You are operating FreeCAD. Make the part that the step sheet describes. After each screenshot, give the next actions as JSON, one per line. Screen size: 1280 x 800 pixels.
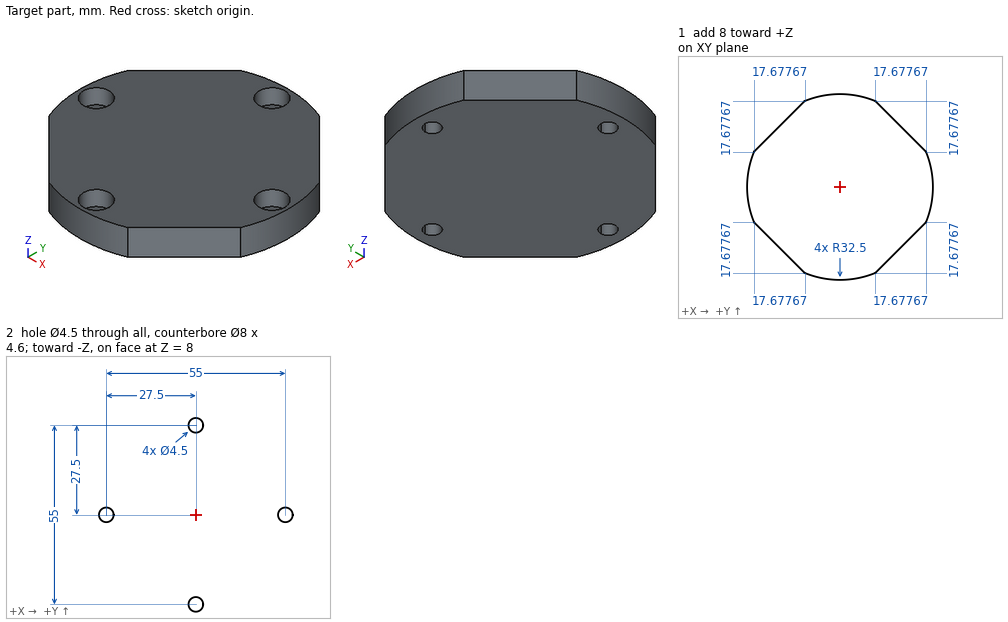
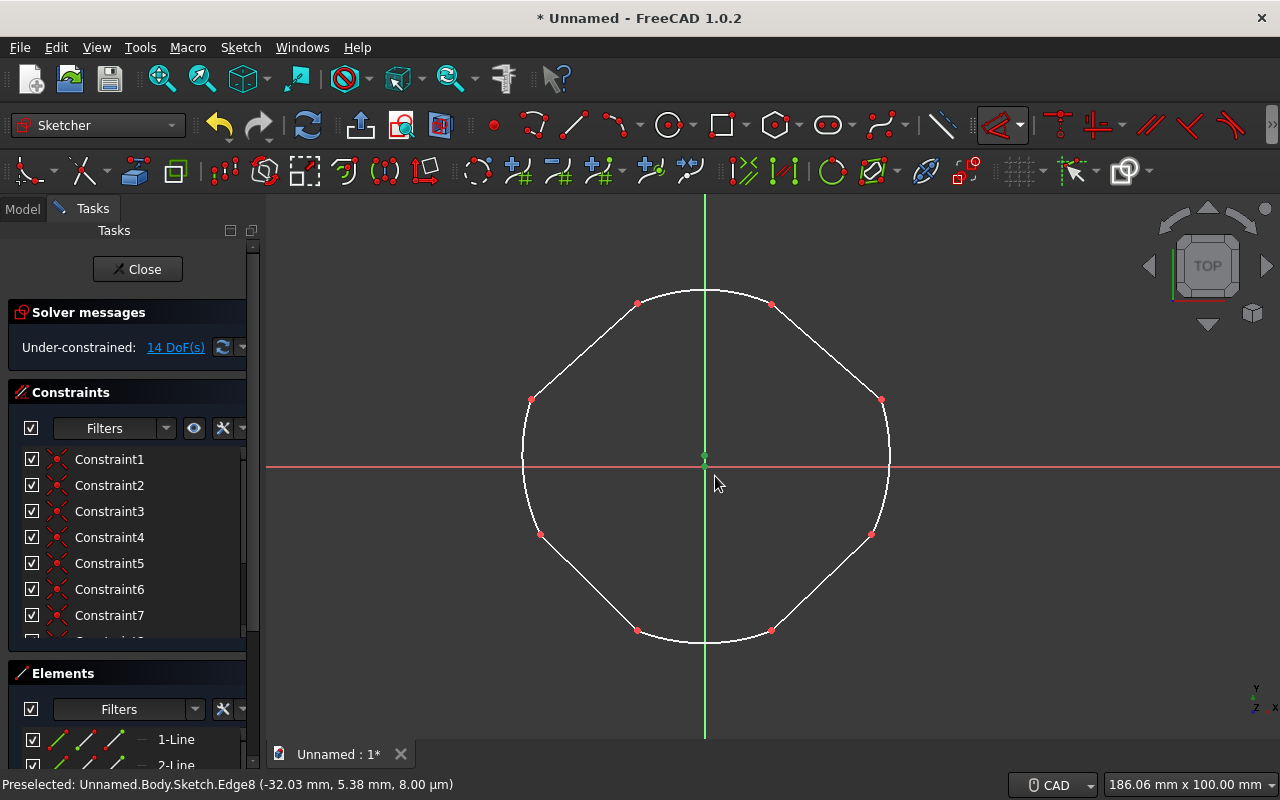
{"action": "left_click", "coordinate": [1058, 126]}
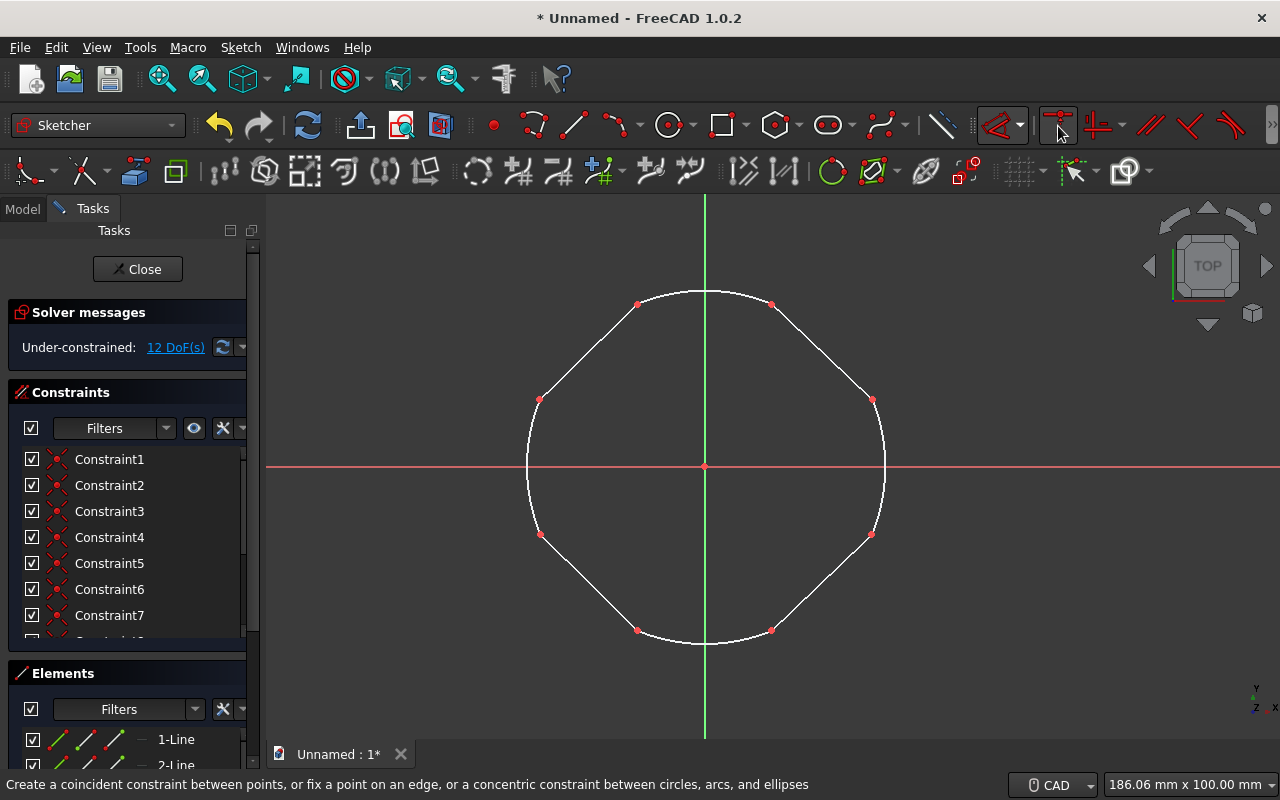
{"action": "left_click", "coordinate": [677, 642]}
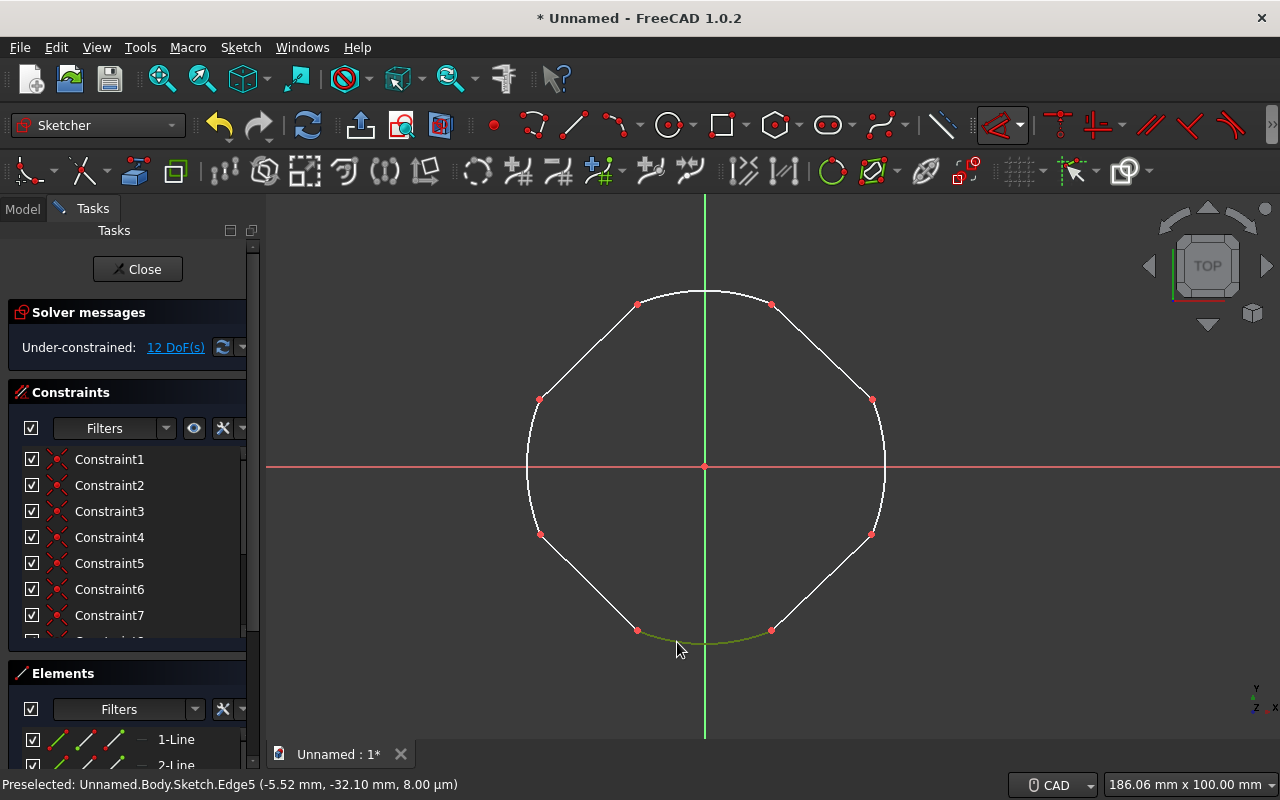
{"action": "left_click", "coordinate": [883, 495]}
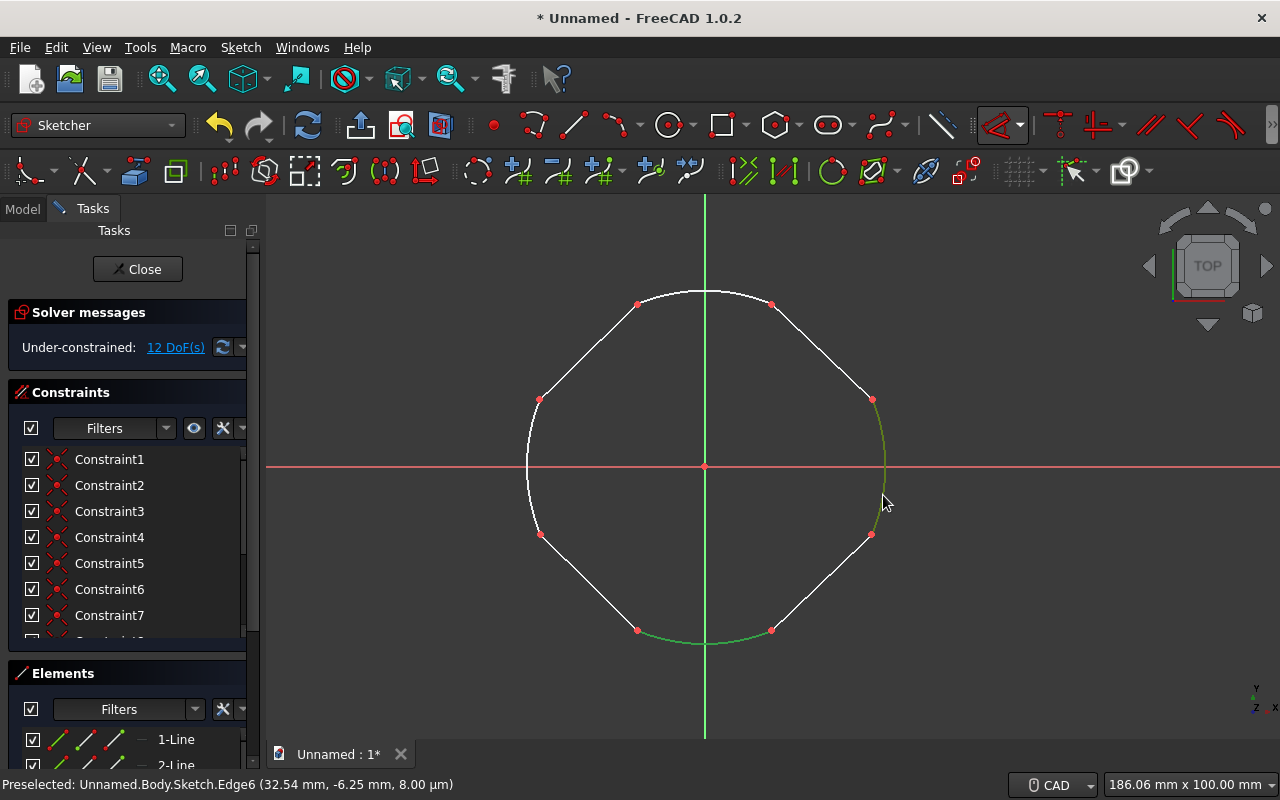
{"action": "left_click", "coordinate": [732, 293]}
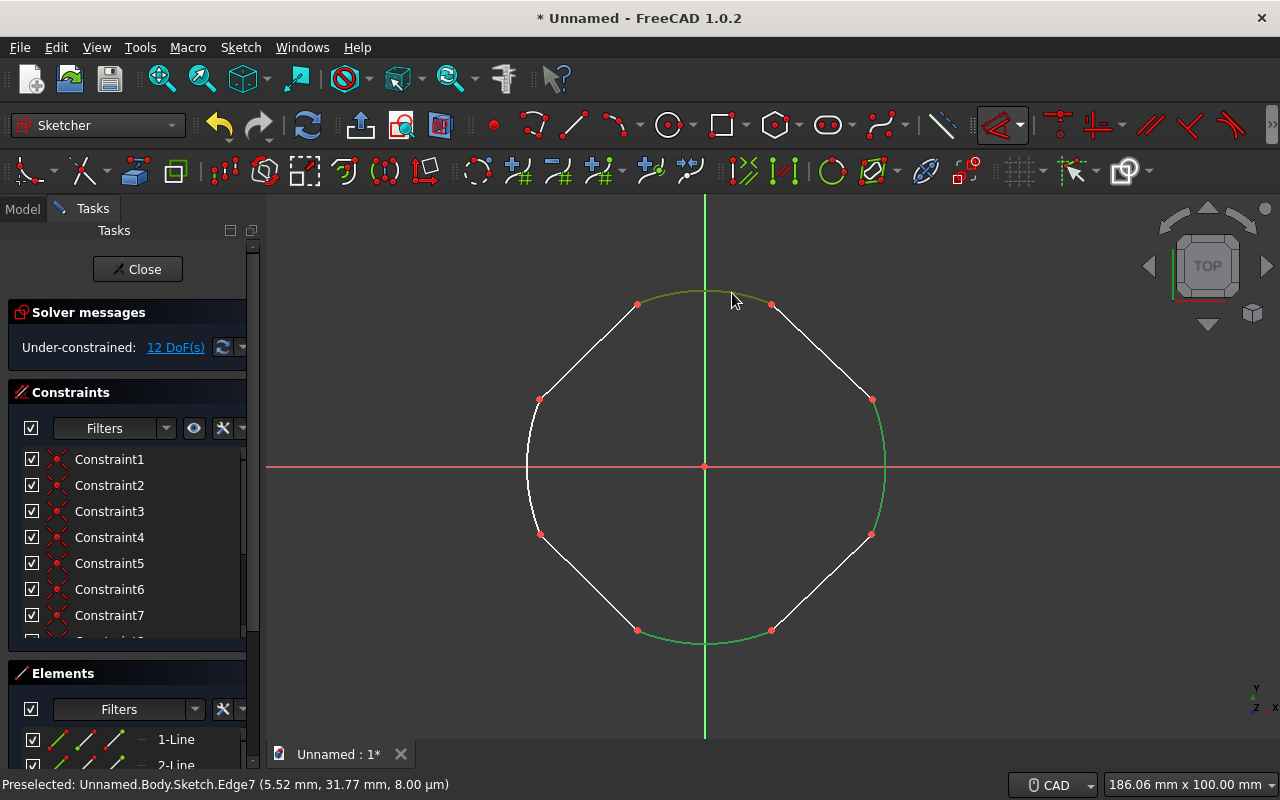
{"action": "left_click", "coordinate": [529, 440]}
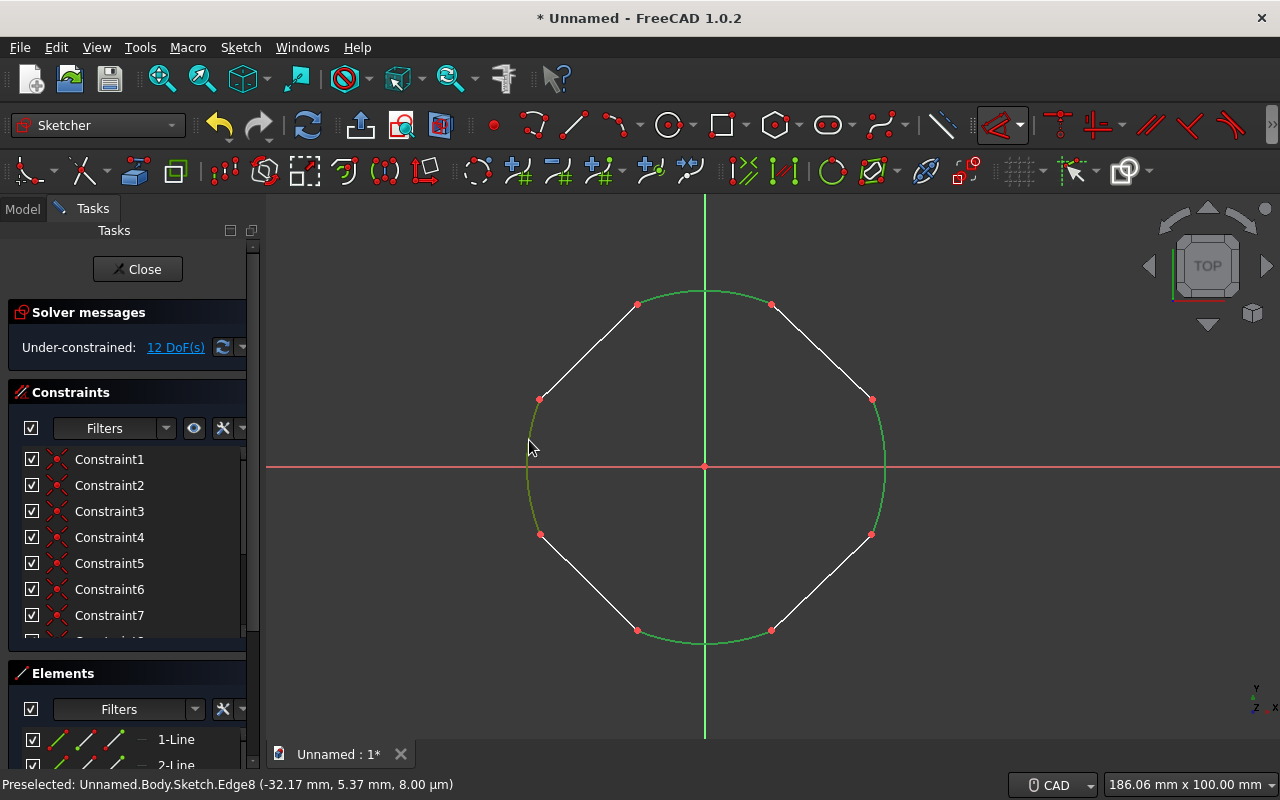
{"action": "key", "text": "e"}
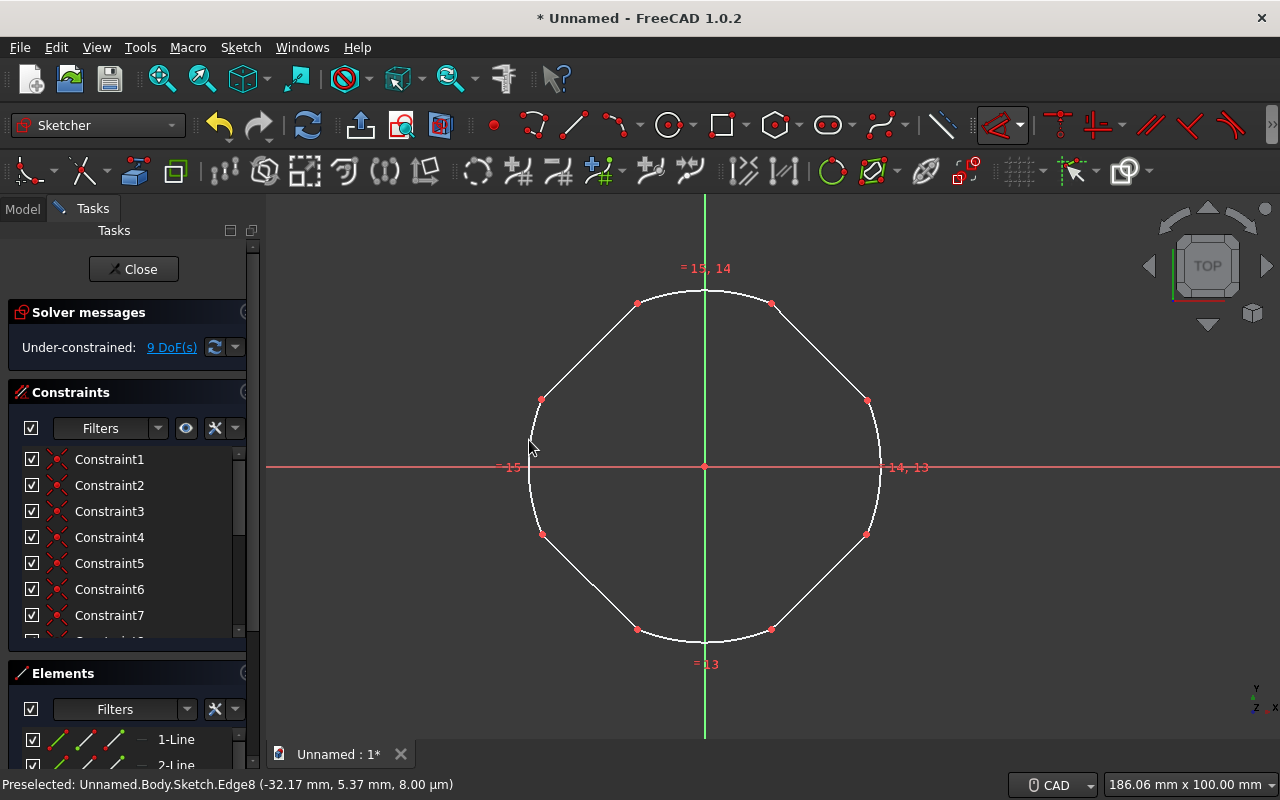
{"action": "left_click", "coordinate": [996, 126]}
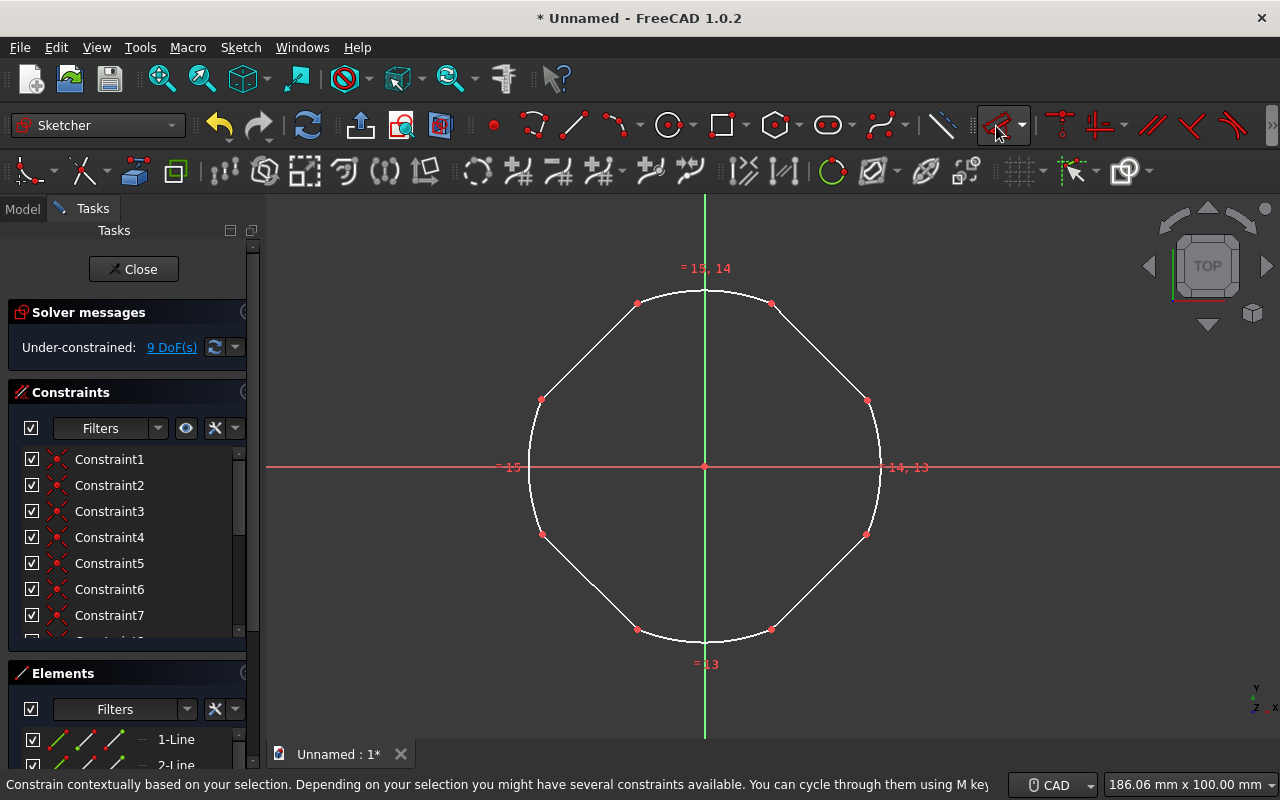
{"action": "left_click", "coordinate": [677, 640]}
{"action": "left_click", "coordinate": [672, 672]}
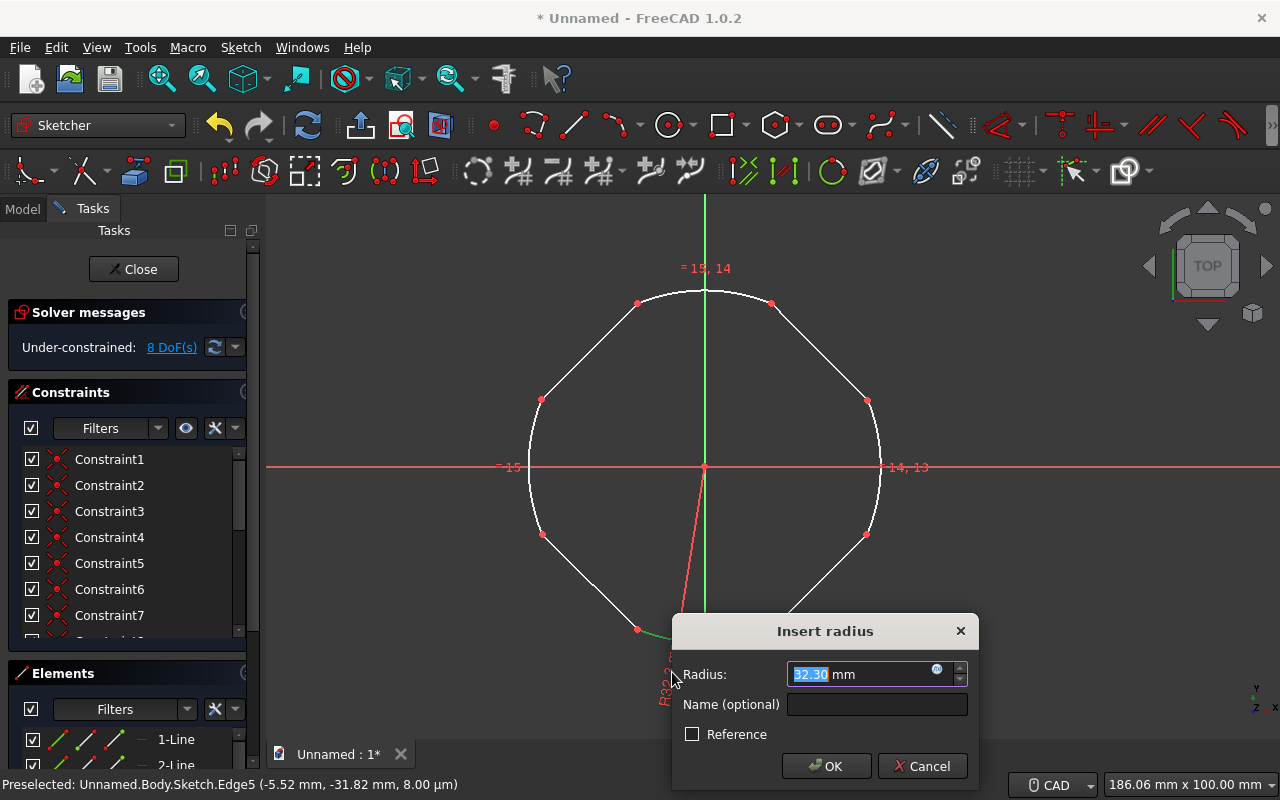
{"action": "type", "text": "32.5"}
{"action": "key", "text": "Return"}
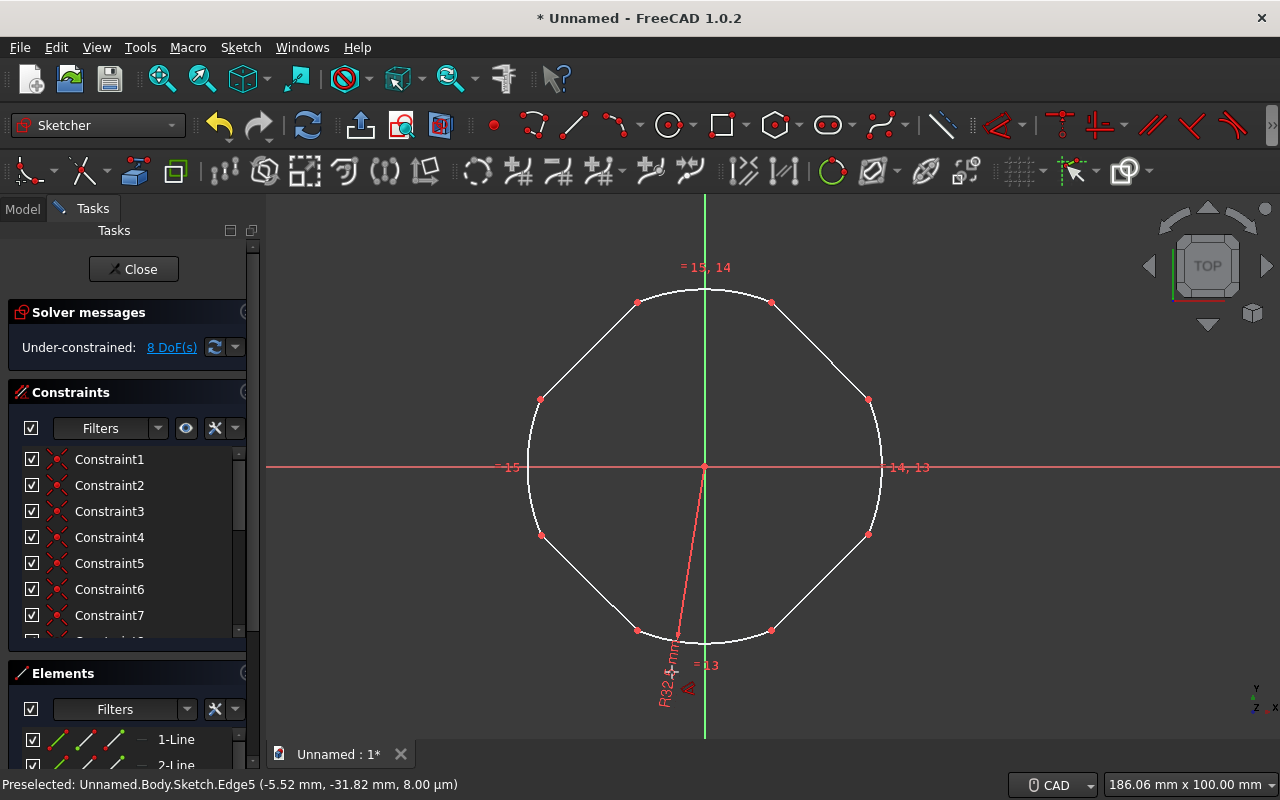
{"action": "left_click", "coordinate": [570, 564]}
{"action": "left_click", "coordinate": [590, 664]}